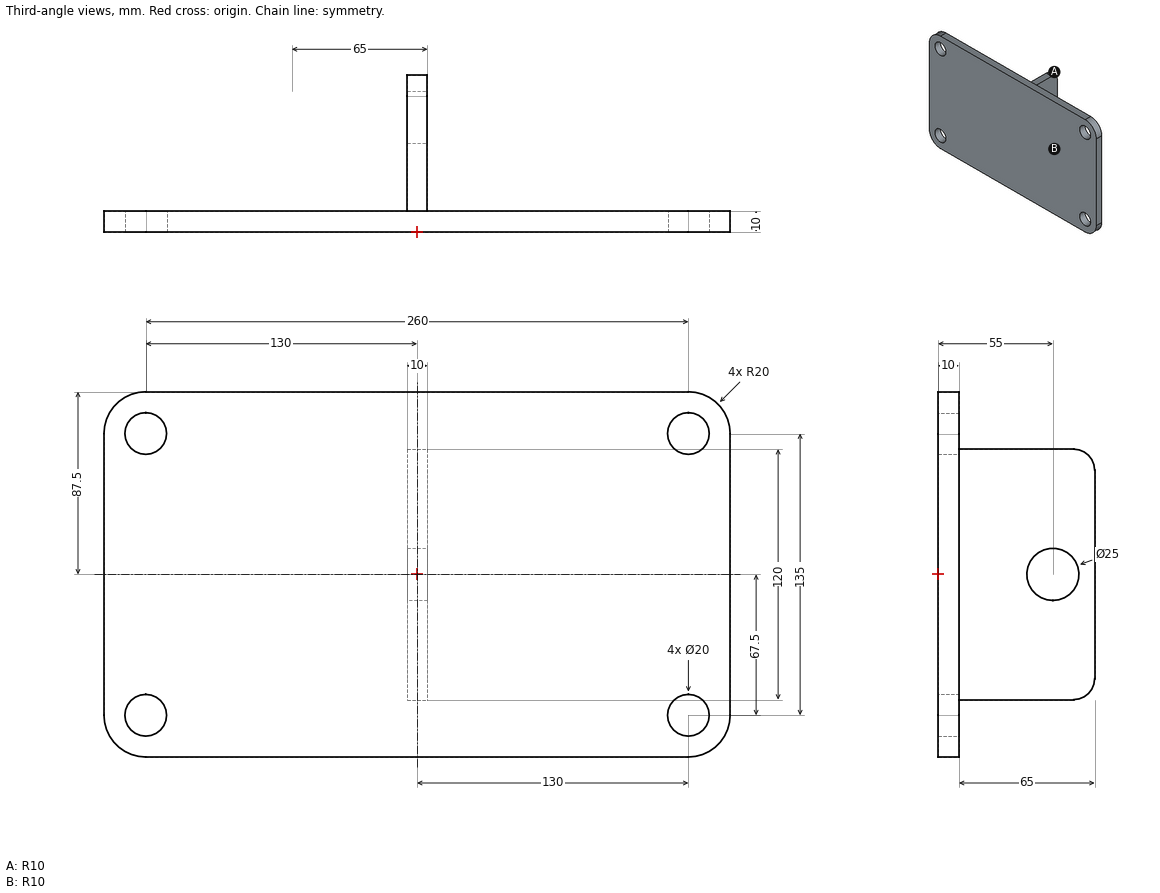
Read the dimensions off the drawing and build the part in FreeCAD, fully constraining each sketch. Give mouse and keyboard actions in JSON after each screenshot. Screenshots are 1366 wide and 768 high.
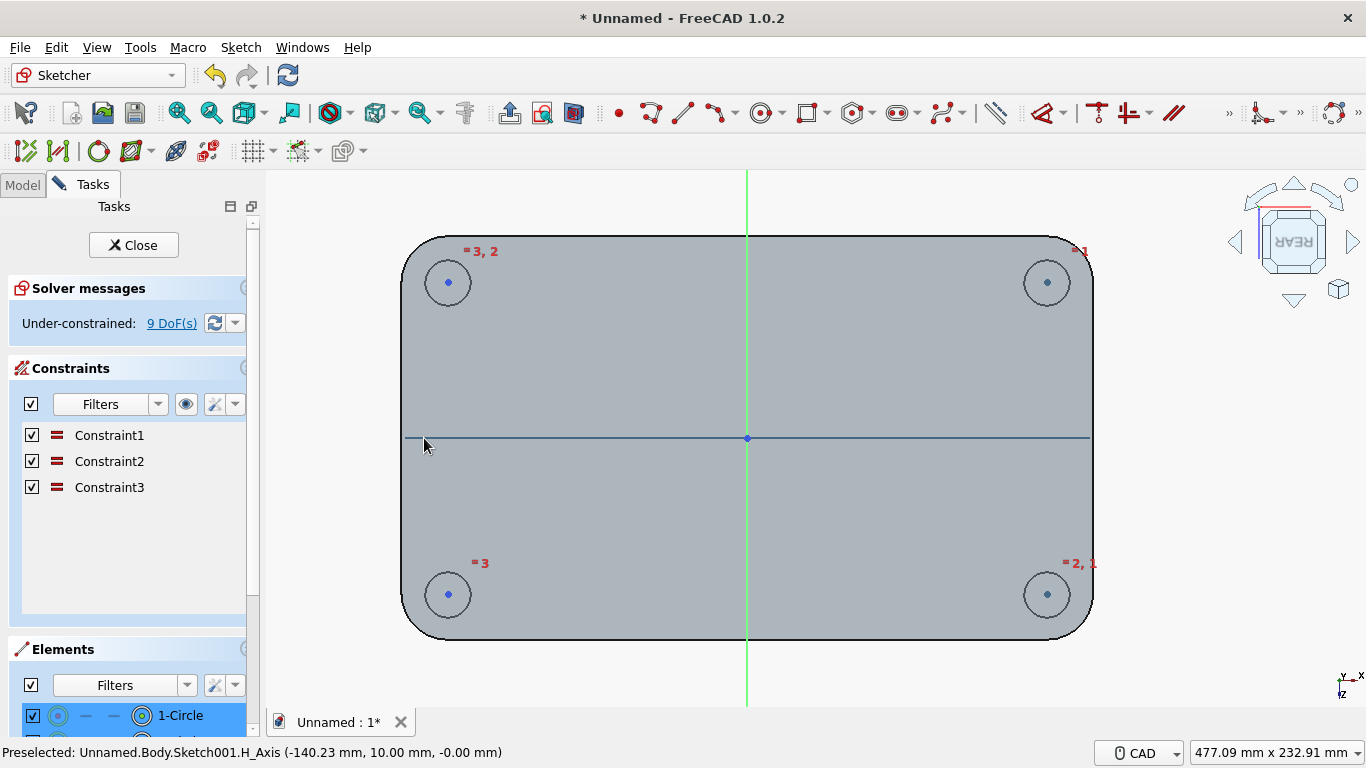
{"action": "key", "text": "s"}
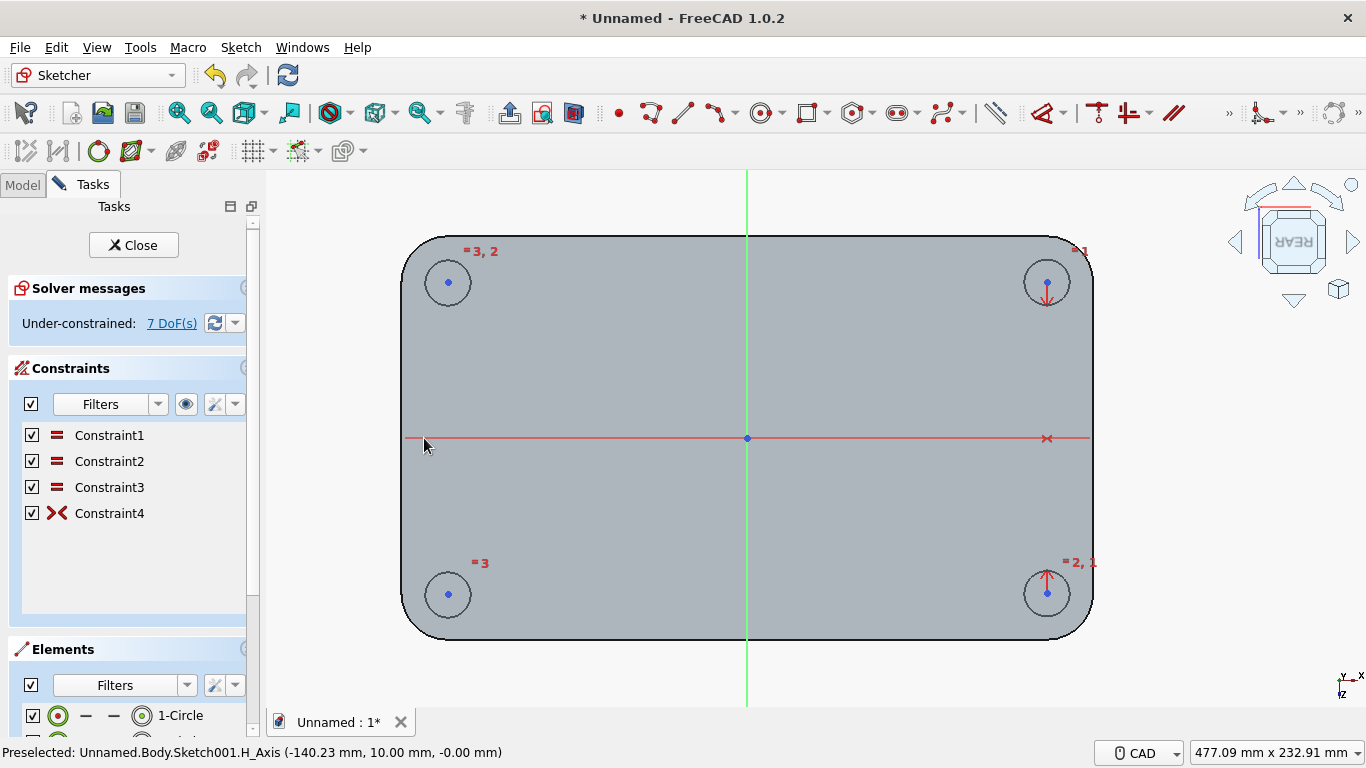
{"action": "left_click", "coordinate": [1047, 282]}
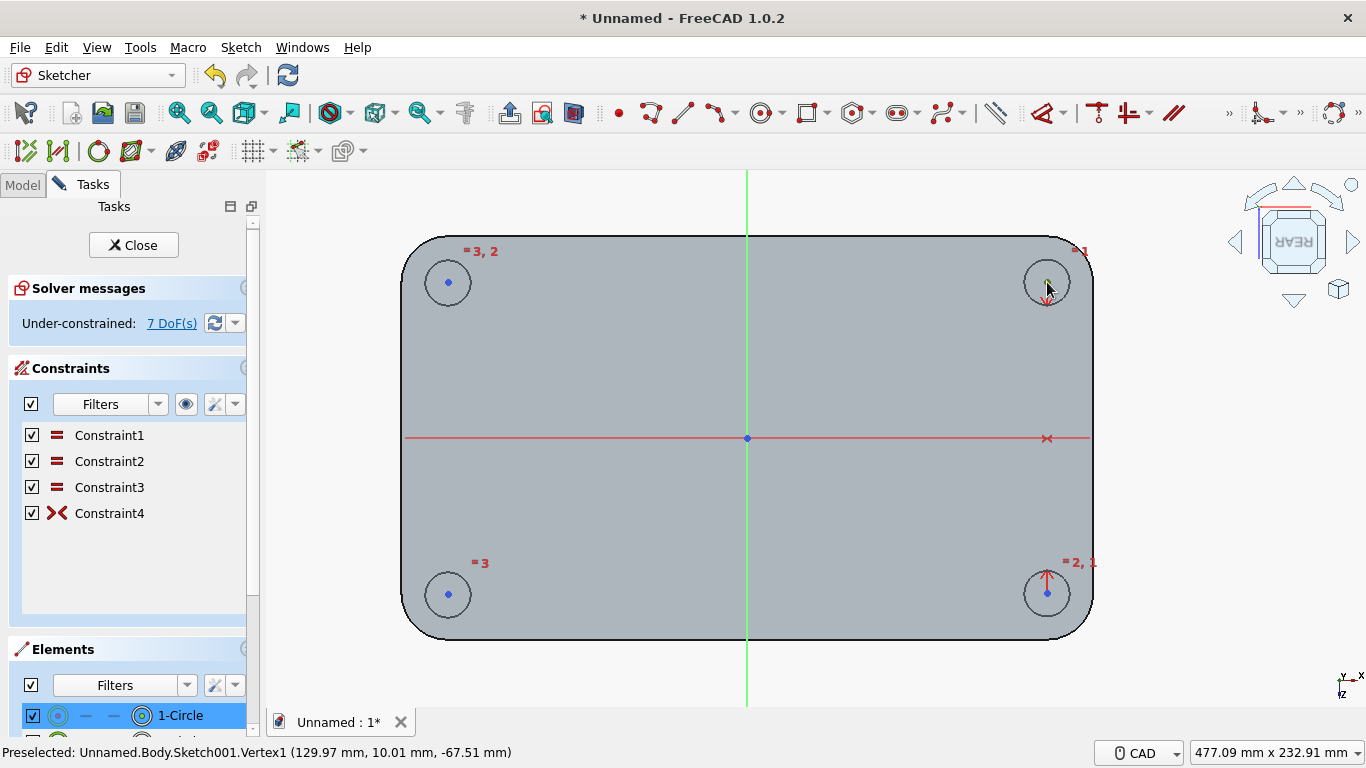
{"action": "left_click", "coordinate": [448, 283]}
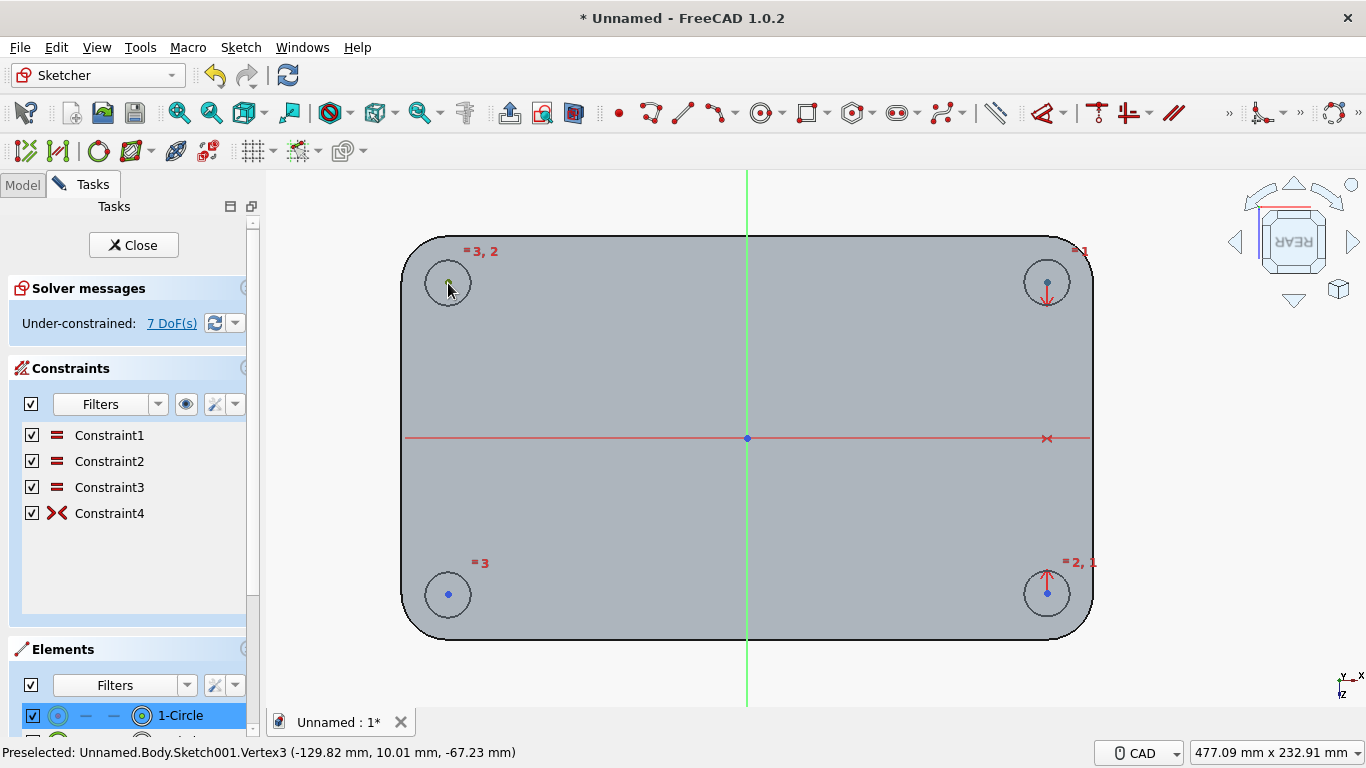
{"action": "left_click", "coordinate": [747, 645]}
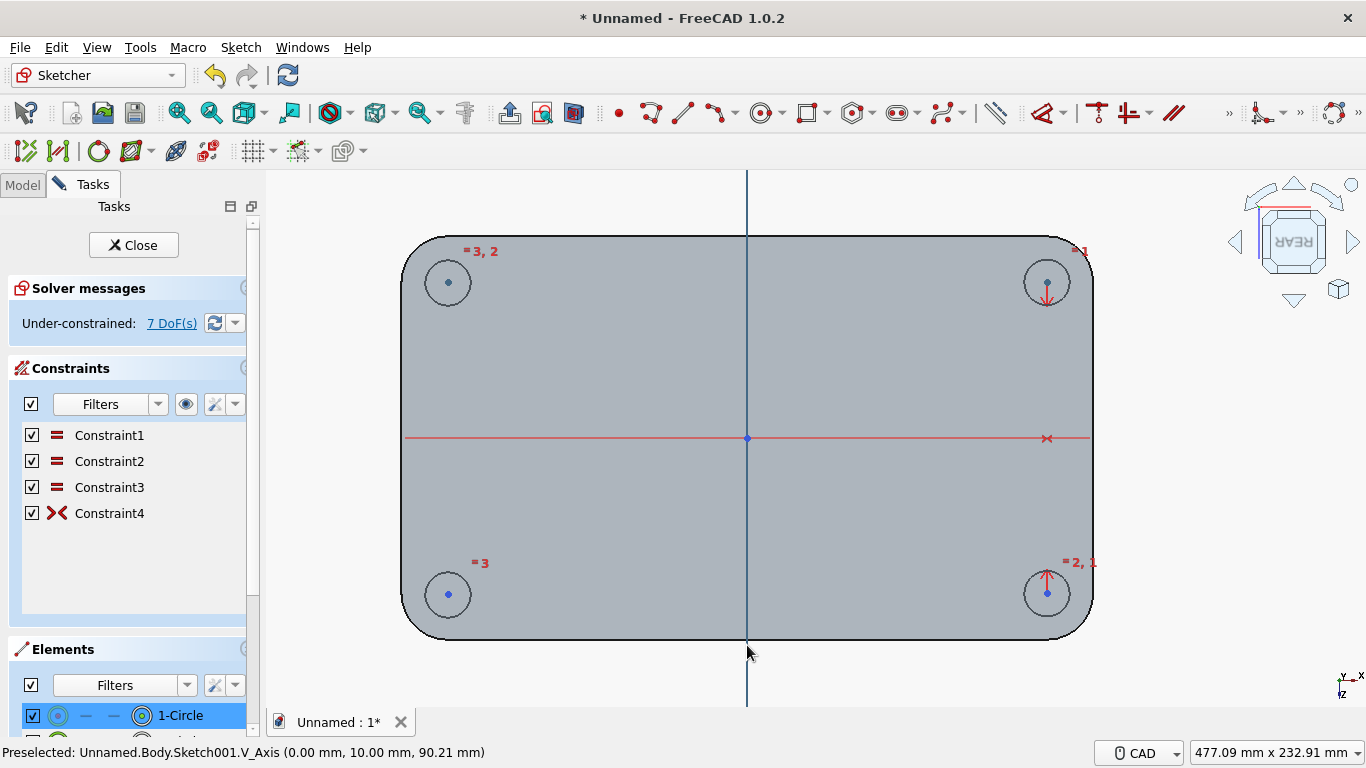
{"action": "key", "text": "s"}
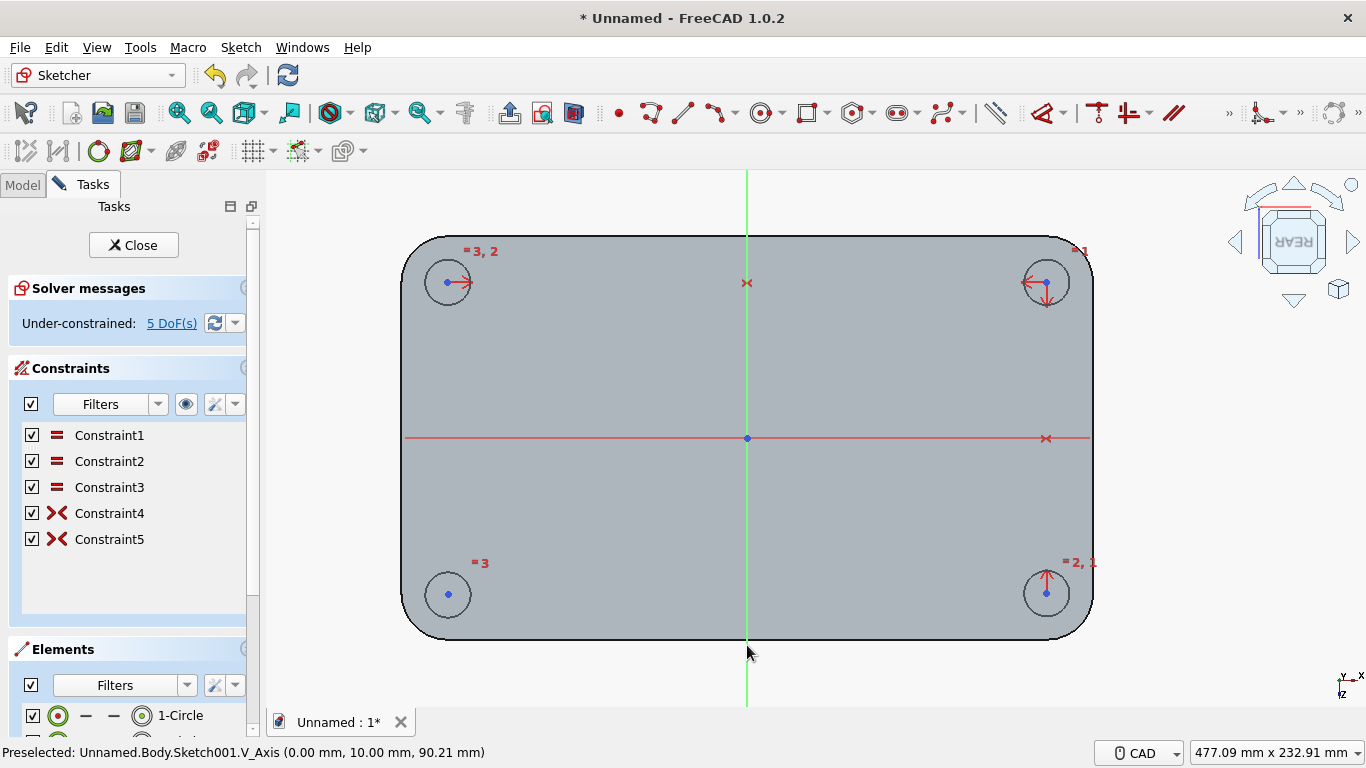
{"action": "left_click", "coordinate": [1047, 594]}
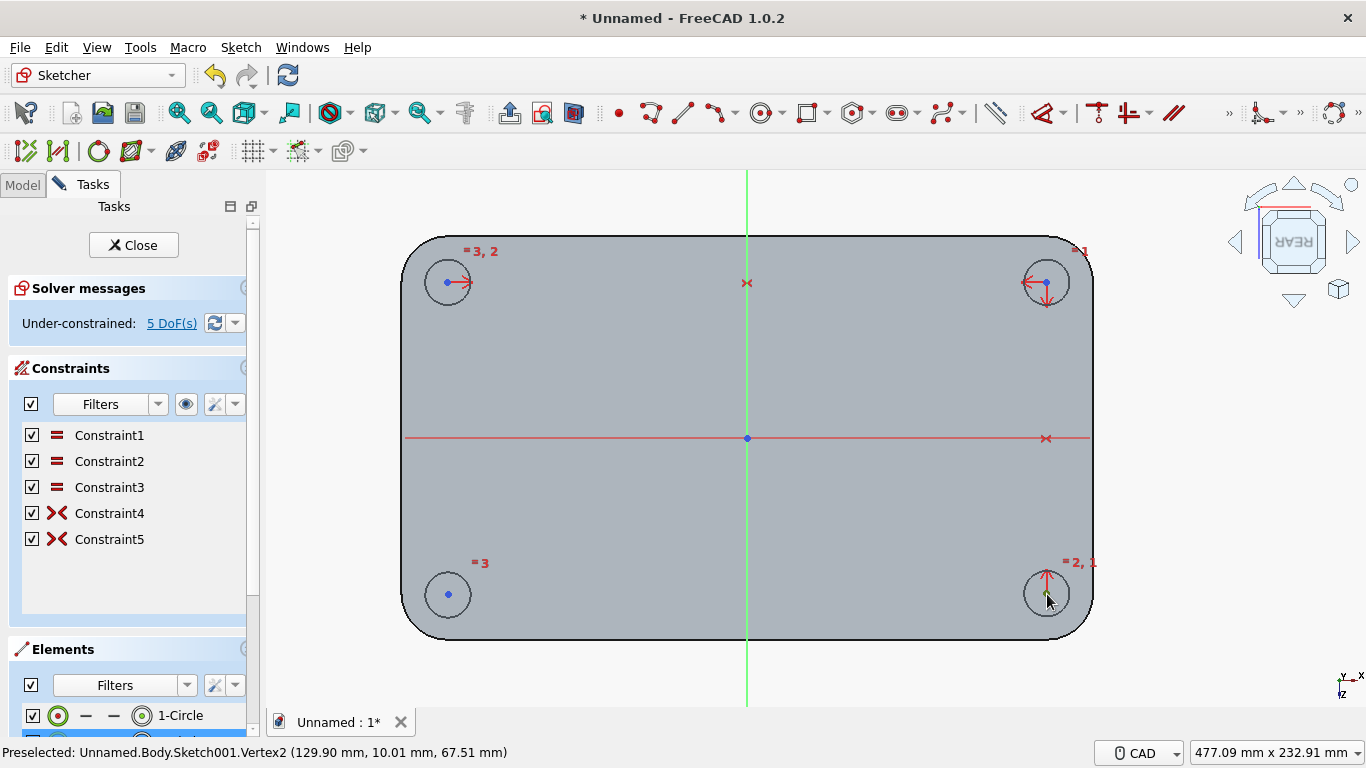
{"action": "left_click", "coordinate": [448, 595]}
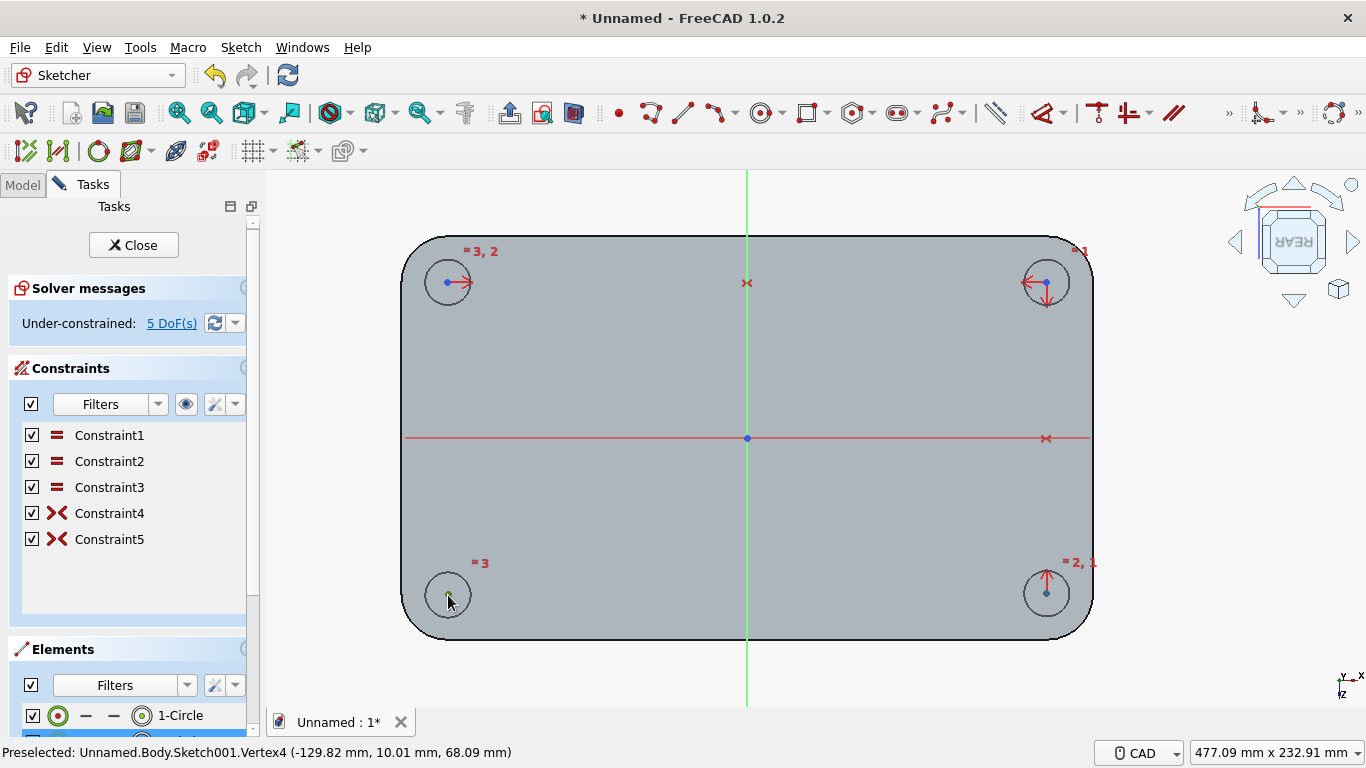
{"action": "left_click", "coordinate": [747, 645]}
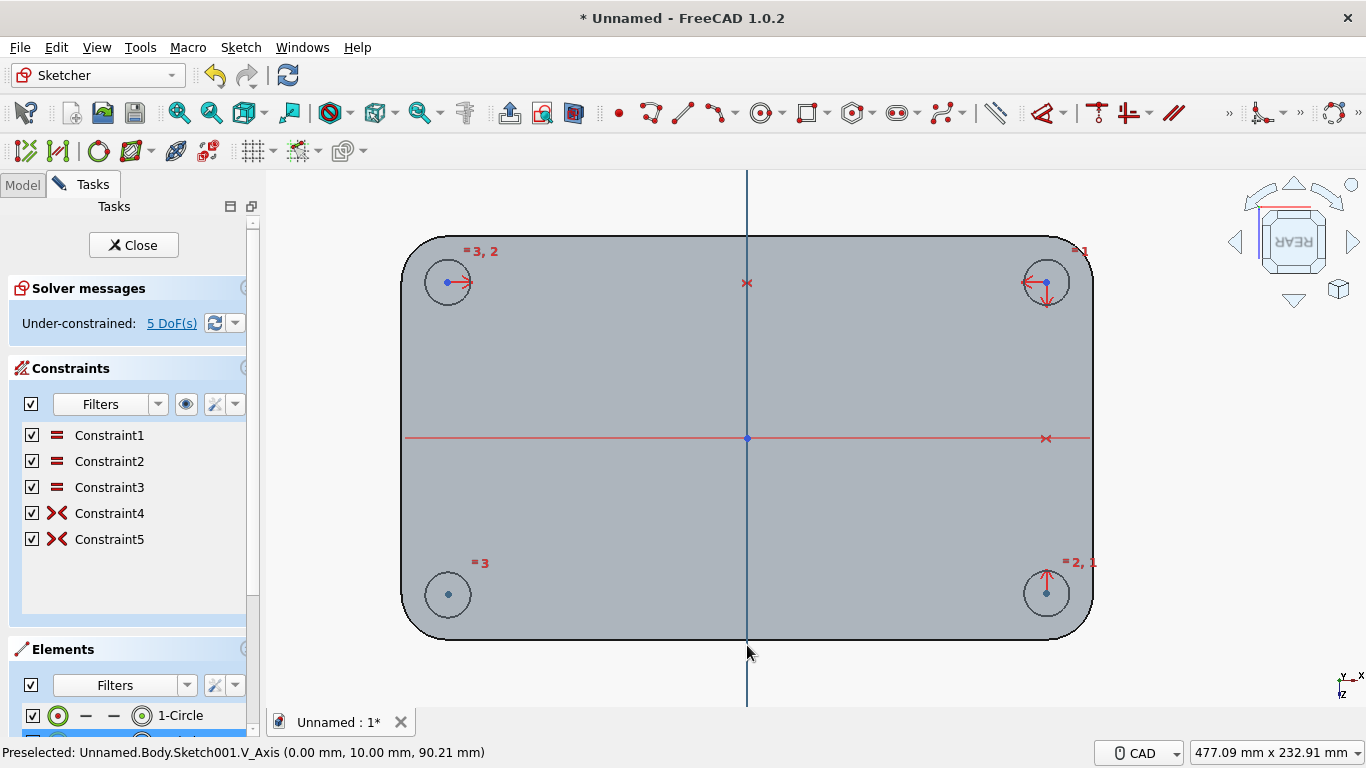
{"action": "key", "text": "s"}